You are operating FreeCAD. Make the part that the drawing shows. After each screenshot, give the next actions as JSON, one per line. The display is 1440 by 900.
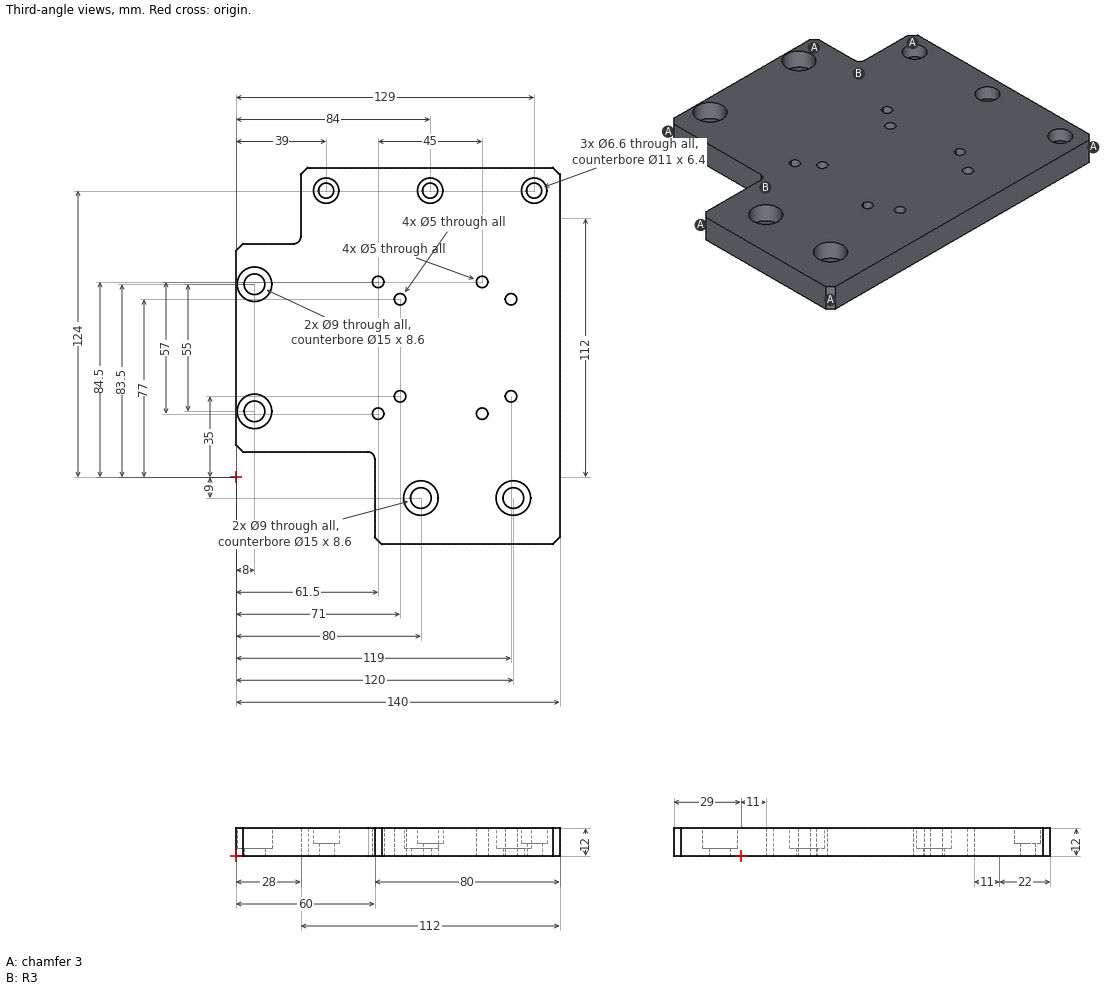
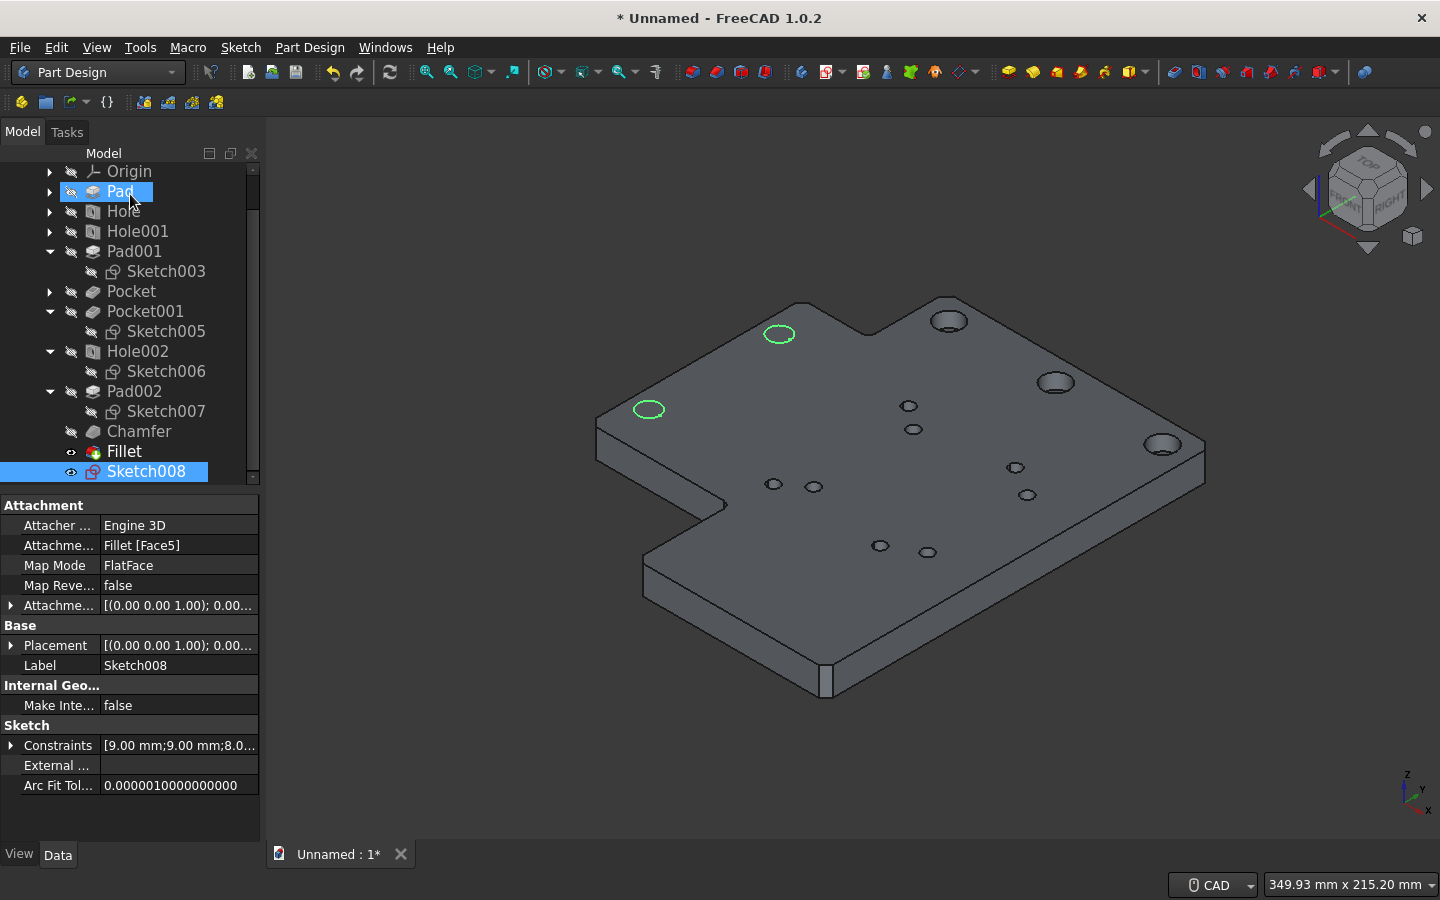
{"action": "left_click", "coordinate": [1200, 72]}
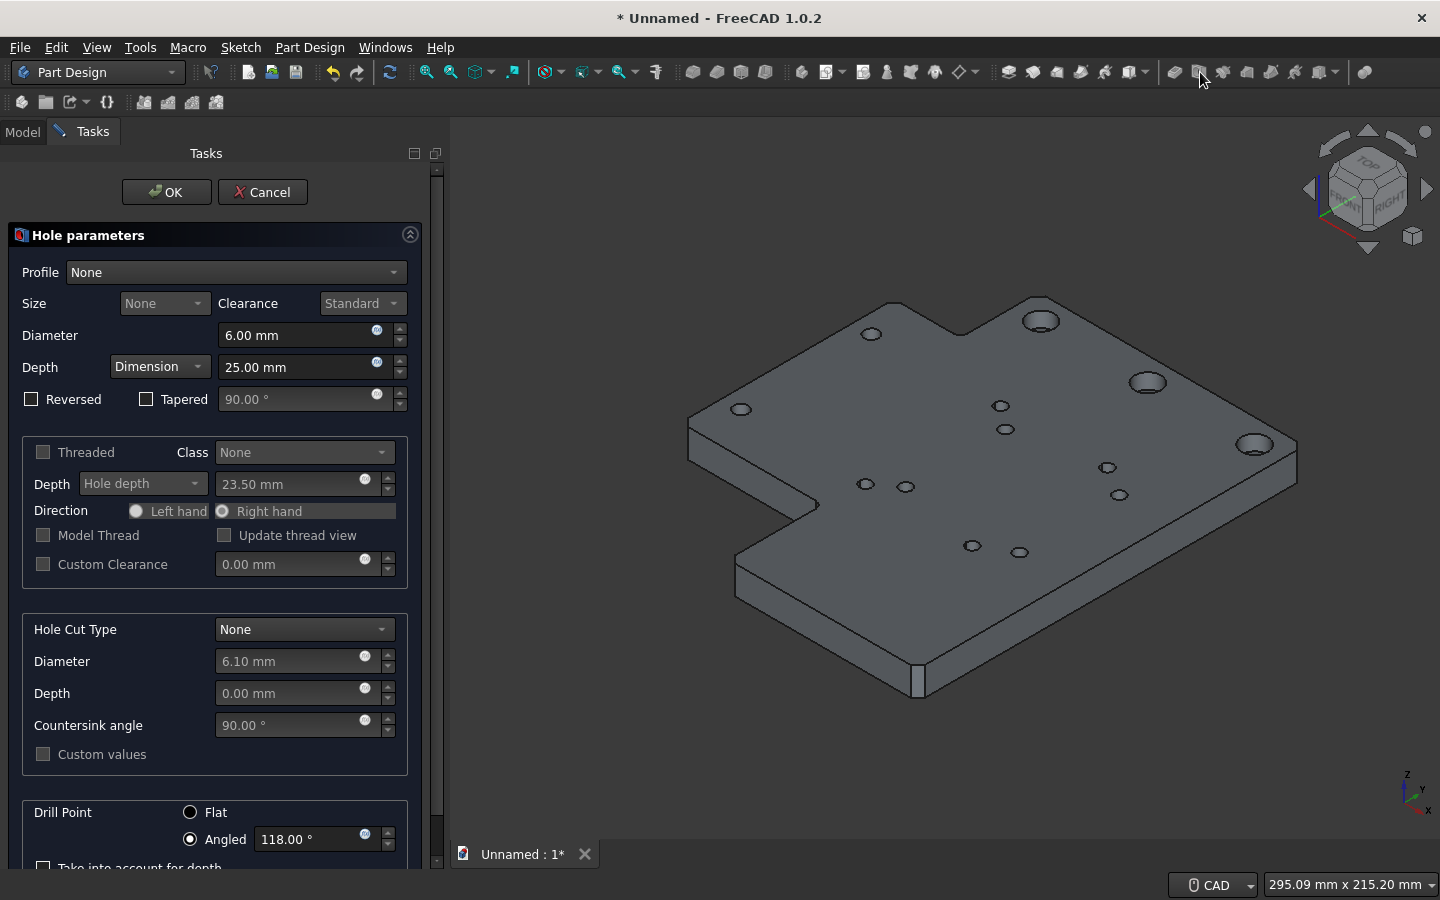
{"action": "triple_click", "coordinate": [305, 335]}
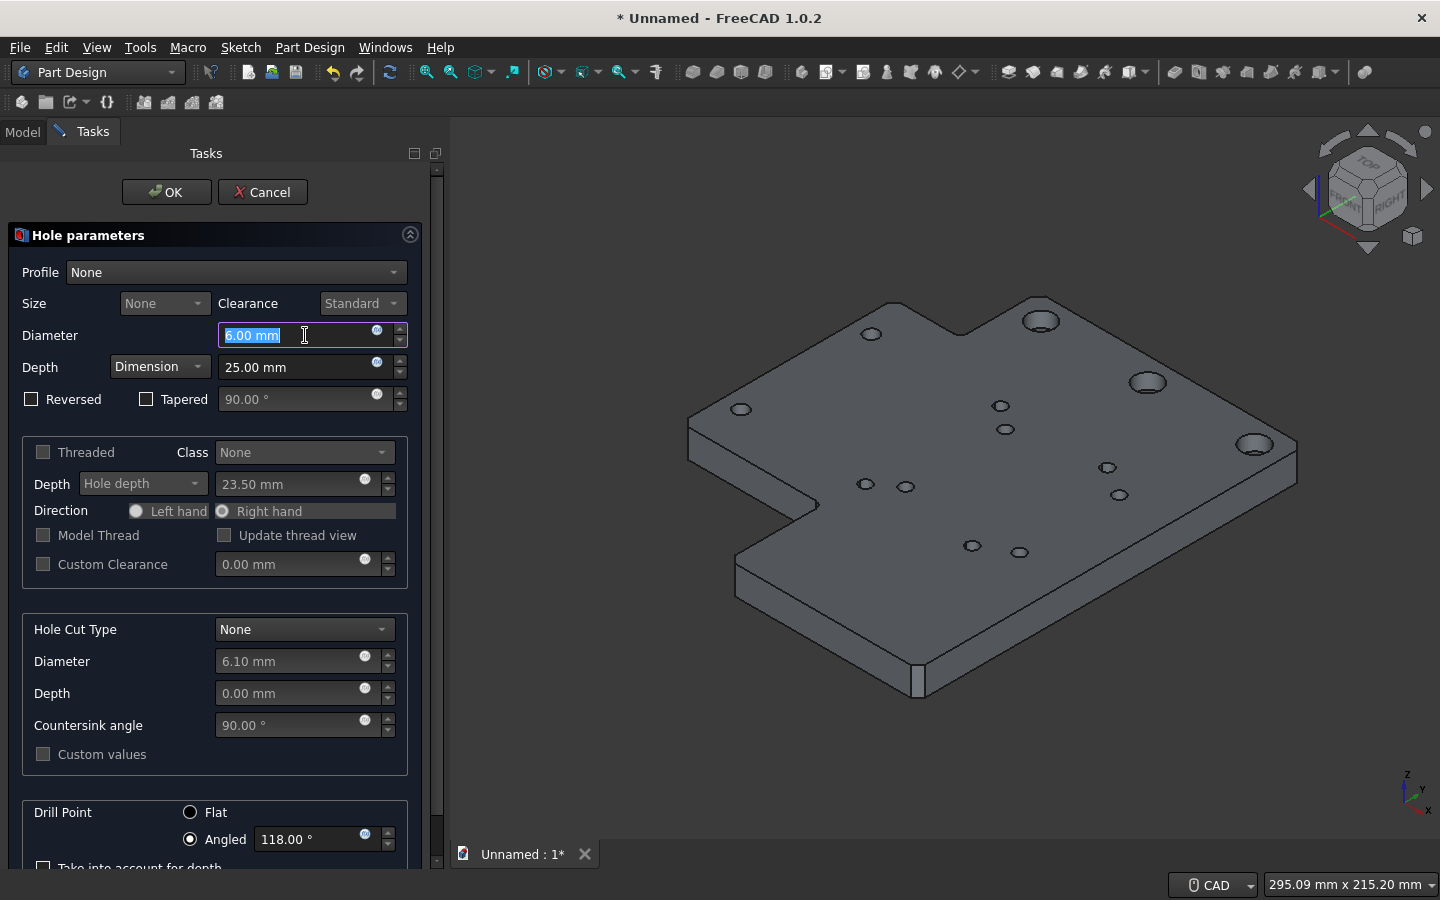
{"action": "type", "text": "9"}
{"action": "key", "text": "Tab"}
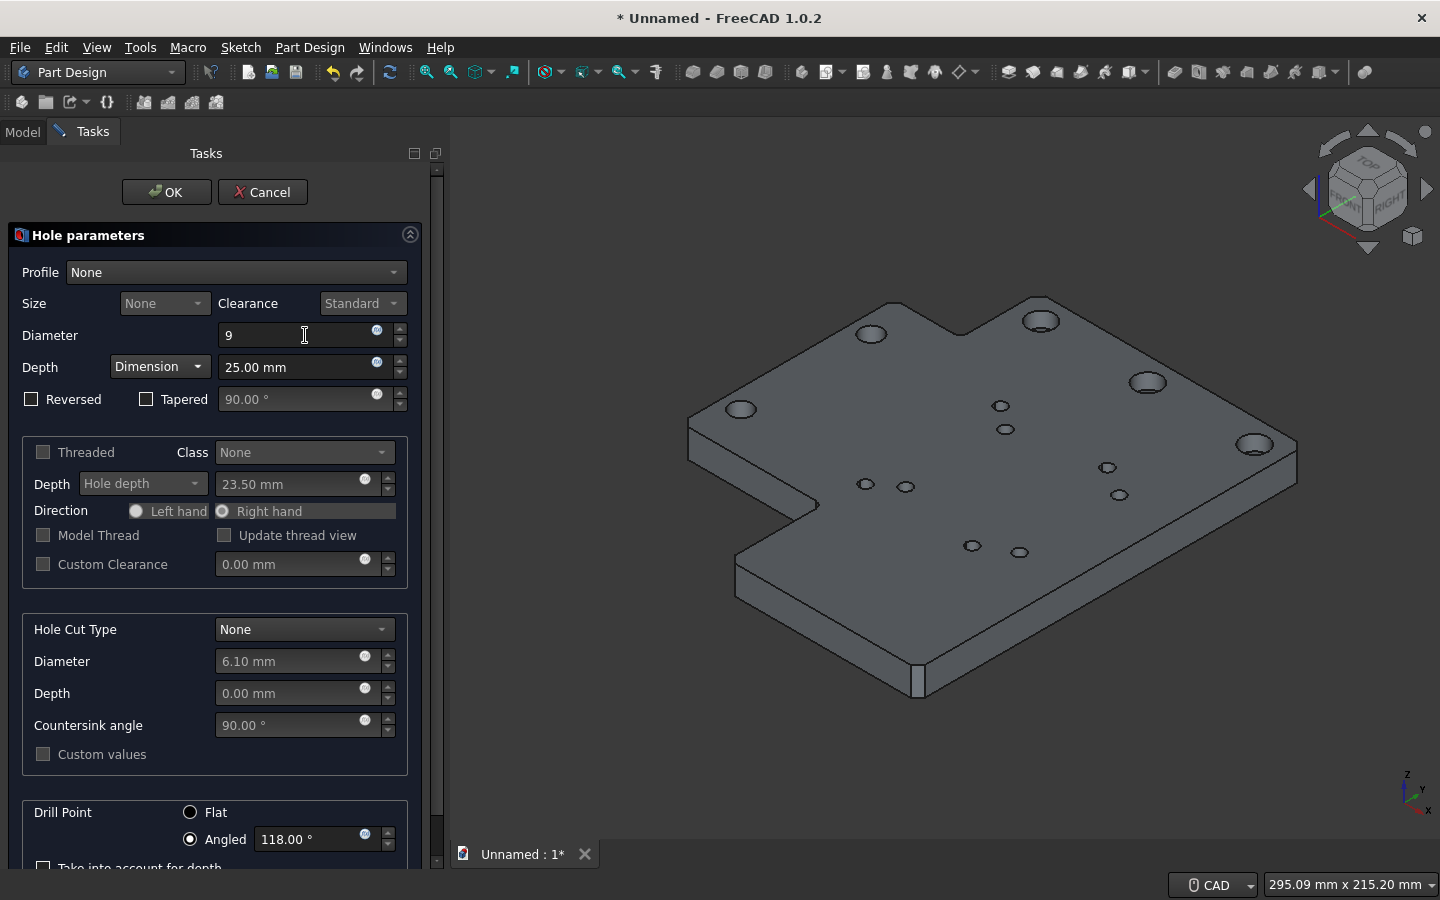
{"action": "left_click", "coordinate": [161, 366]}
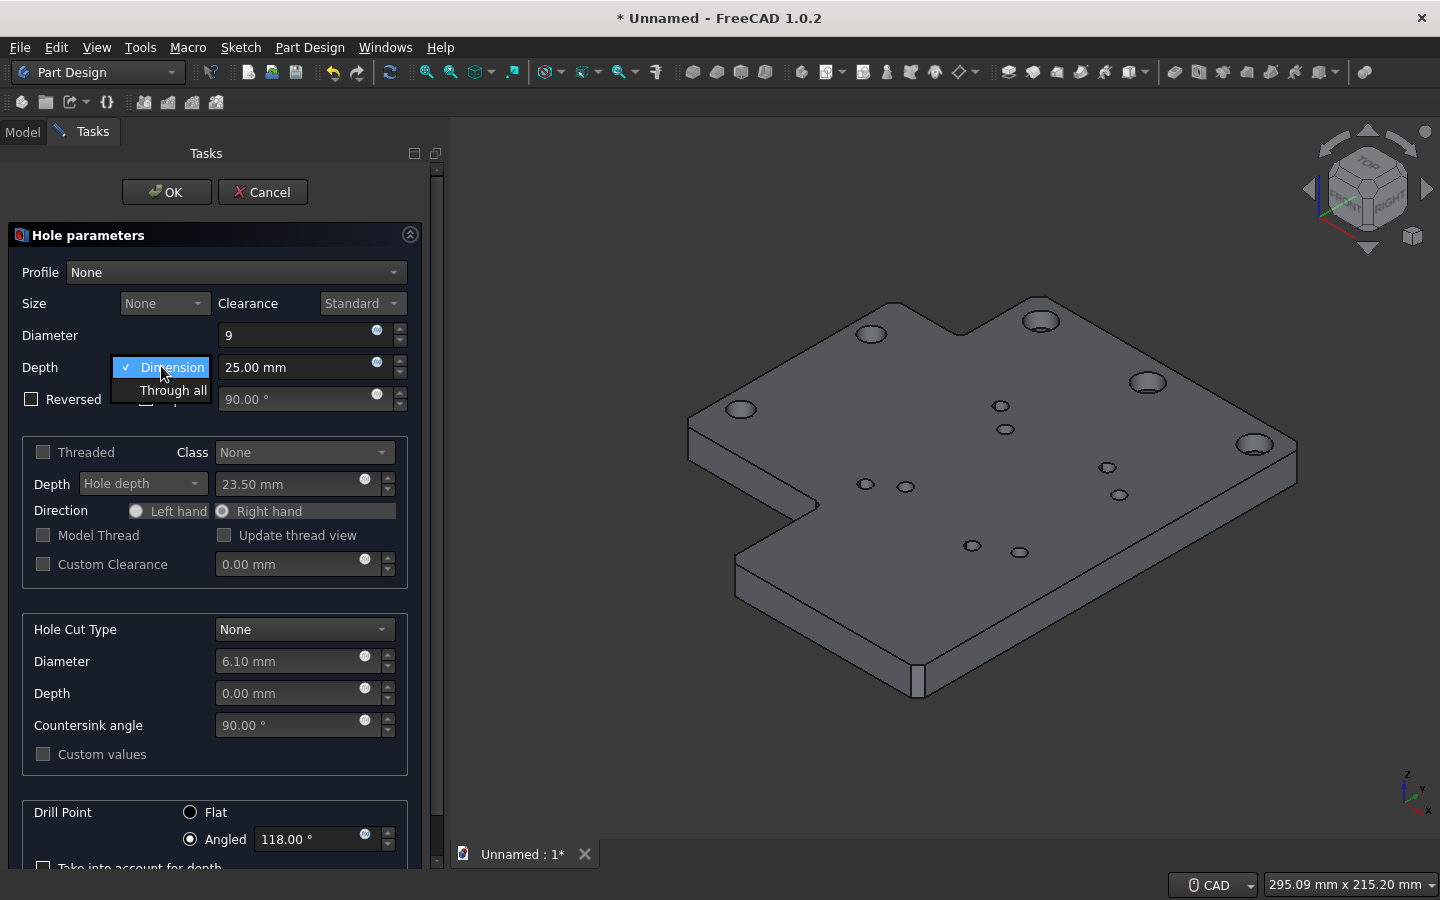
{"action": "left_click", "coordinate": [160, 390]}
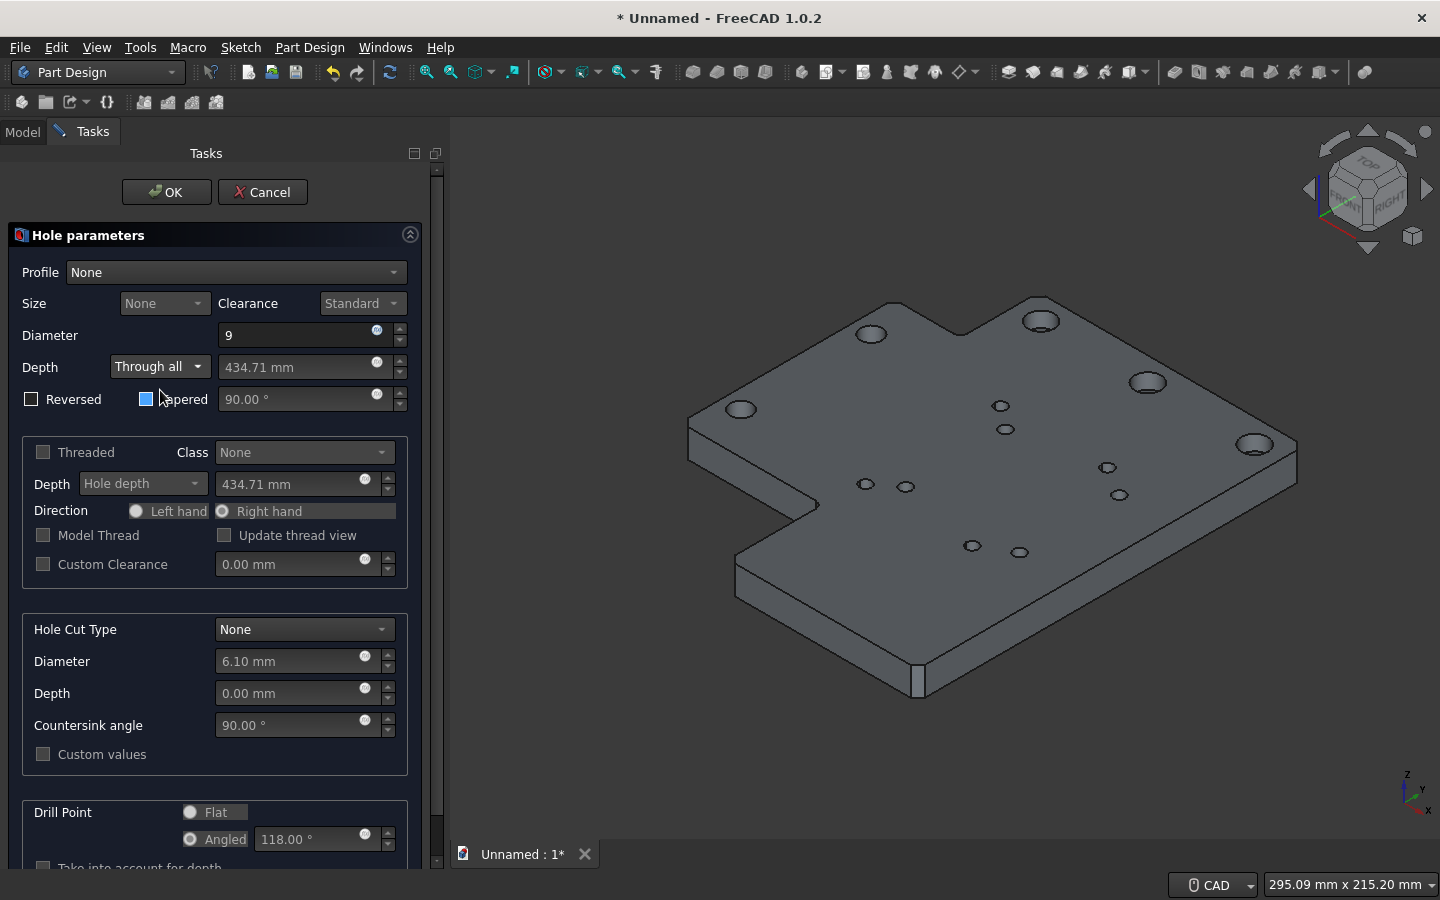
{"action": "left_click", "coordinate": [306, 630]}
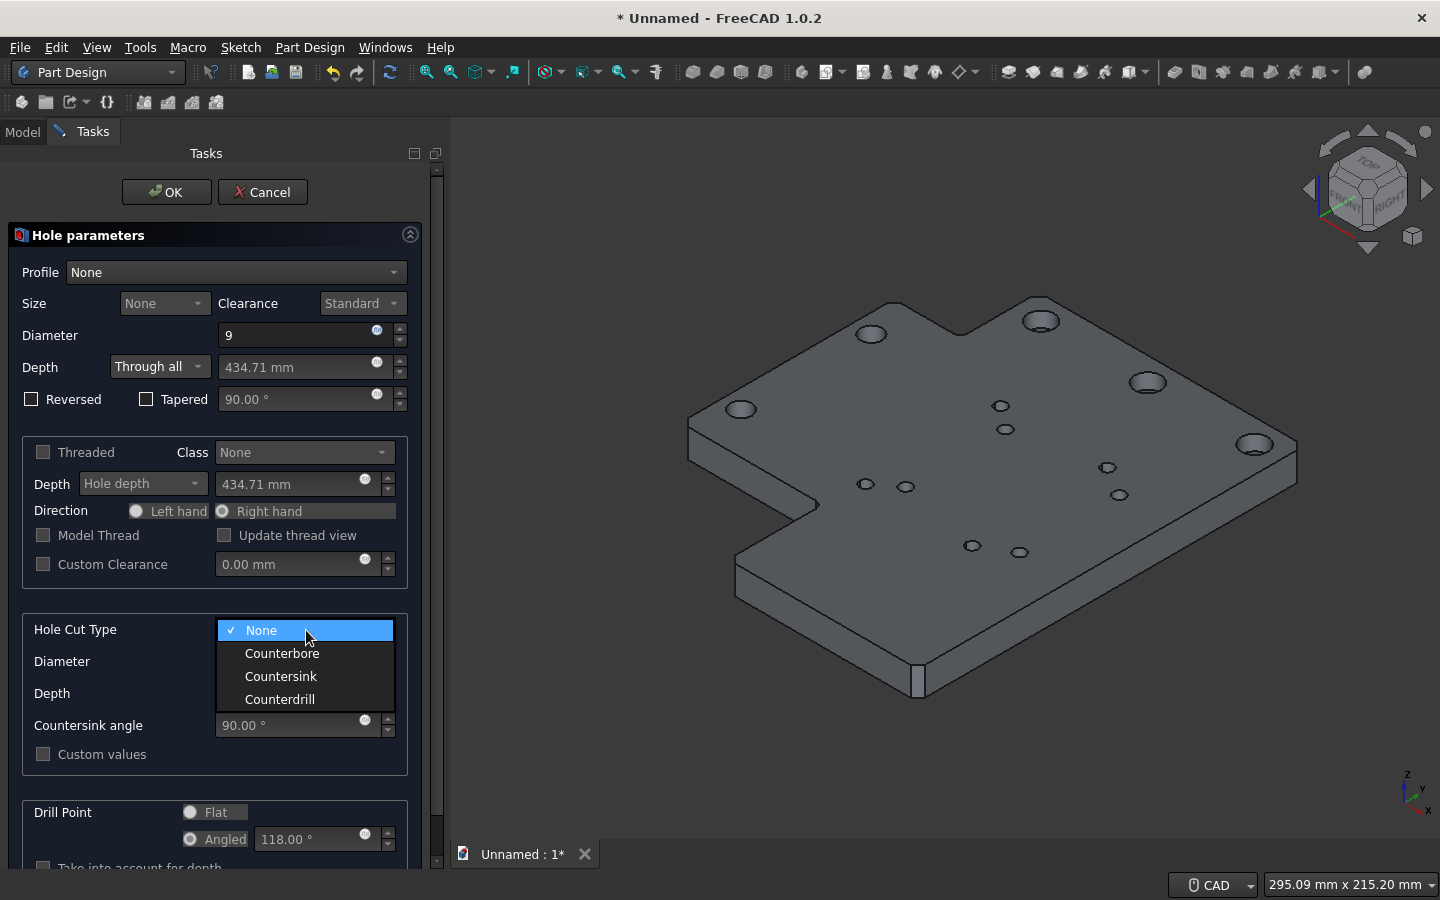
{"action": "left_click", "coordinate": [304, 654]}